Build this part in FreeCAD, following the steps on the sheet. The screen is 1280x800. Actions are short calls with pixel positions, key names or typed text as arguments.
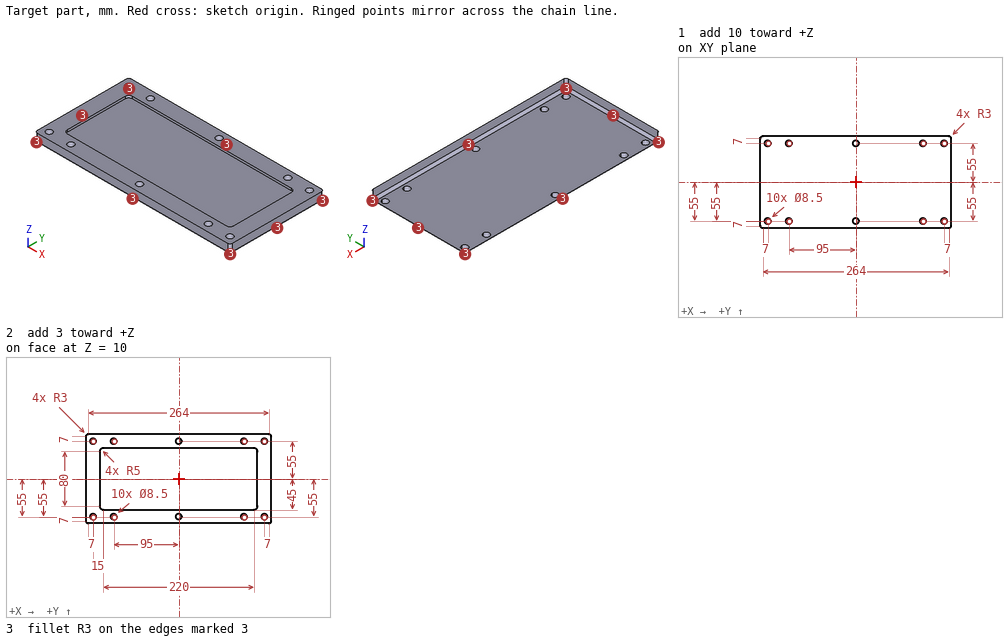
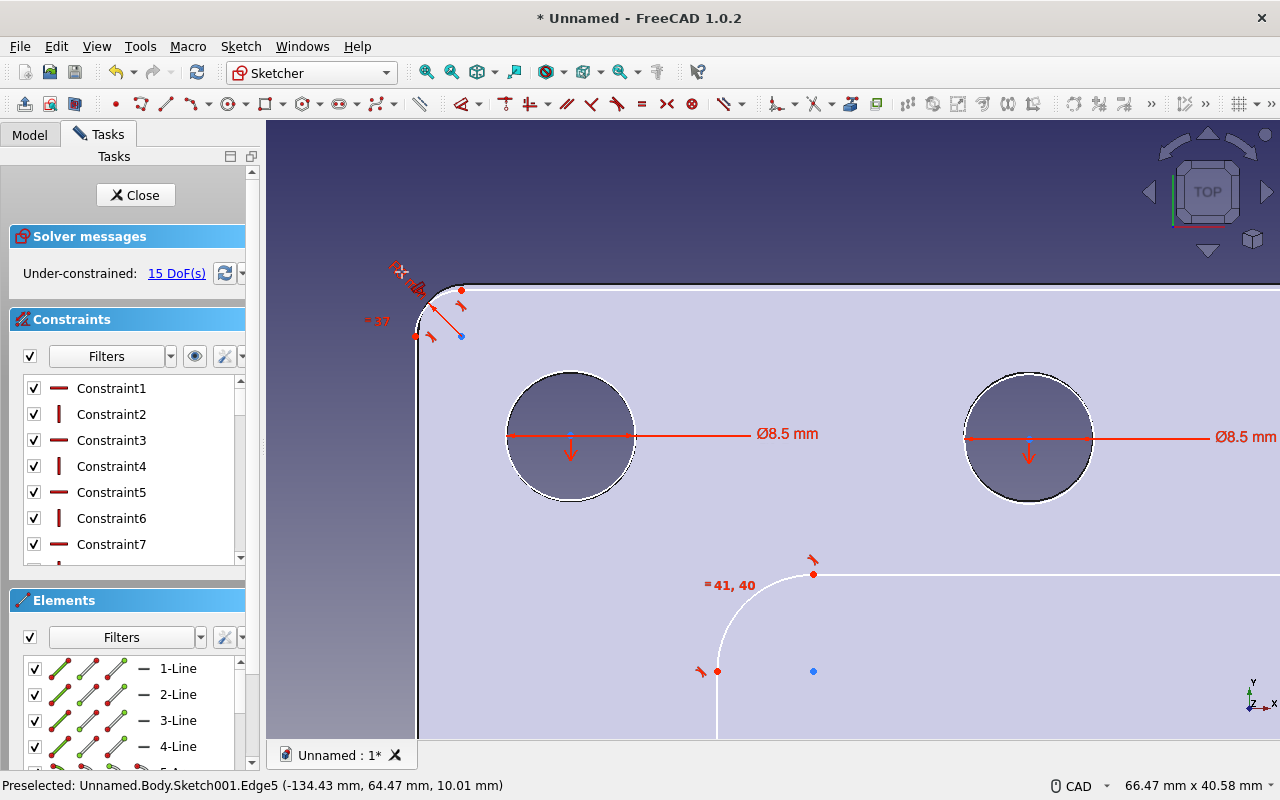
scroll(427, 297, down, 10)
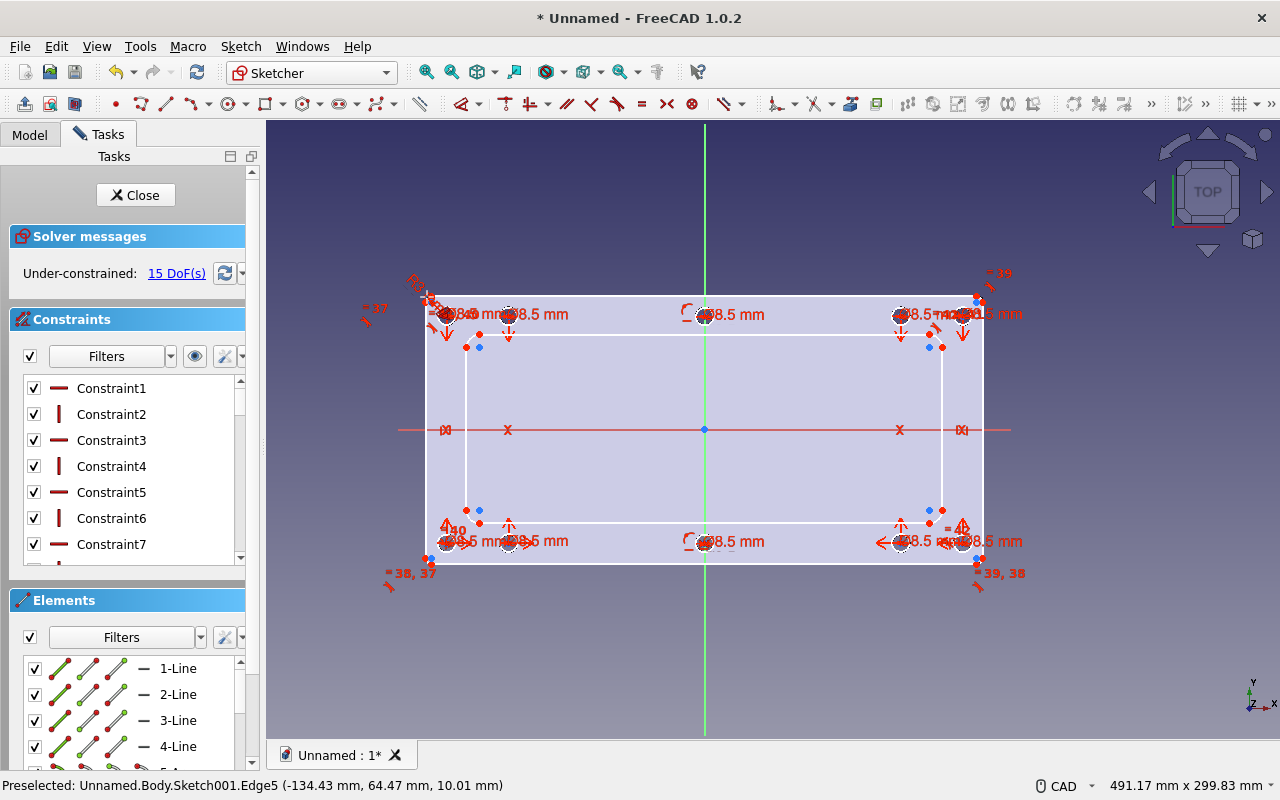
scroll(468, 516, up, 7)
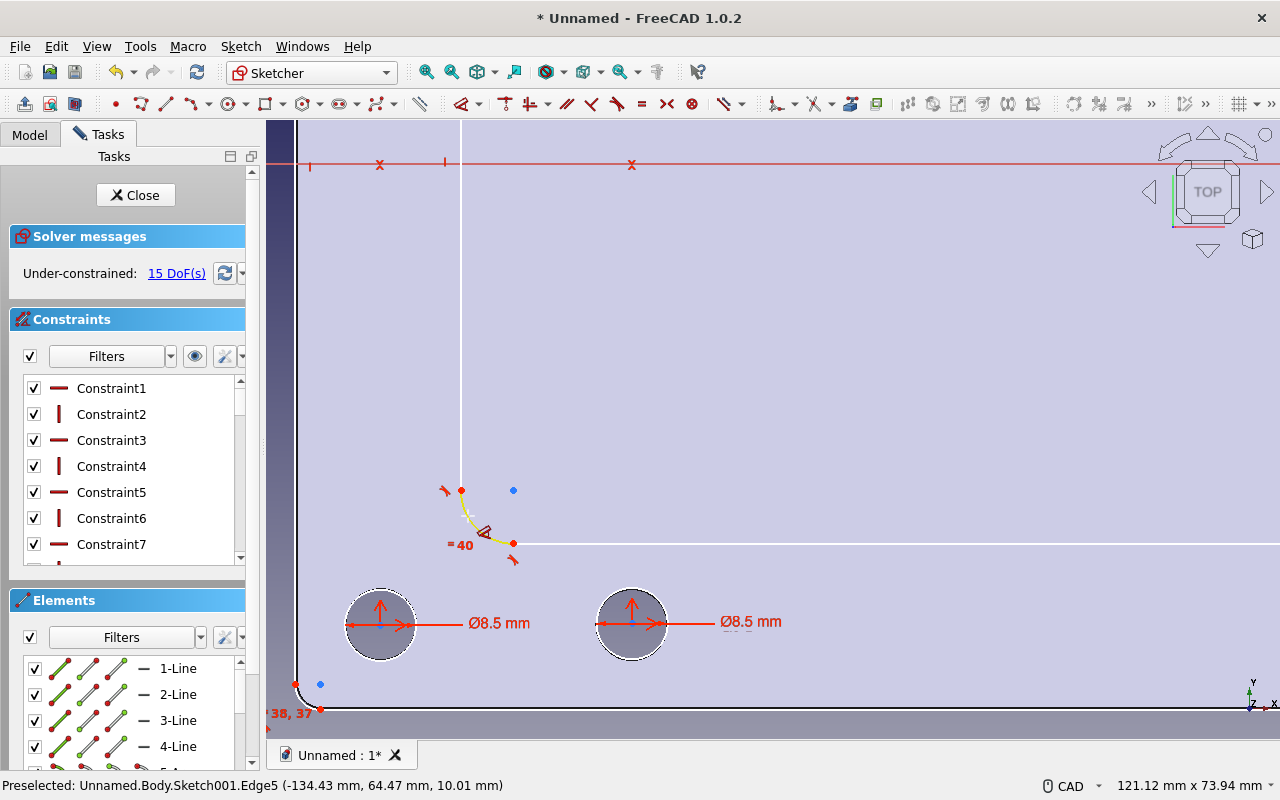
click(467, 515)
click(439, 530)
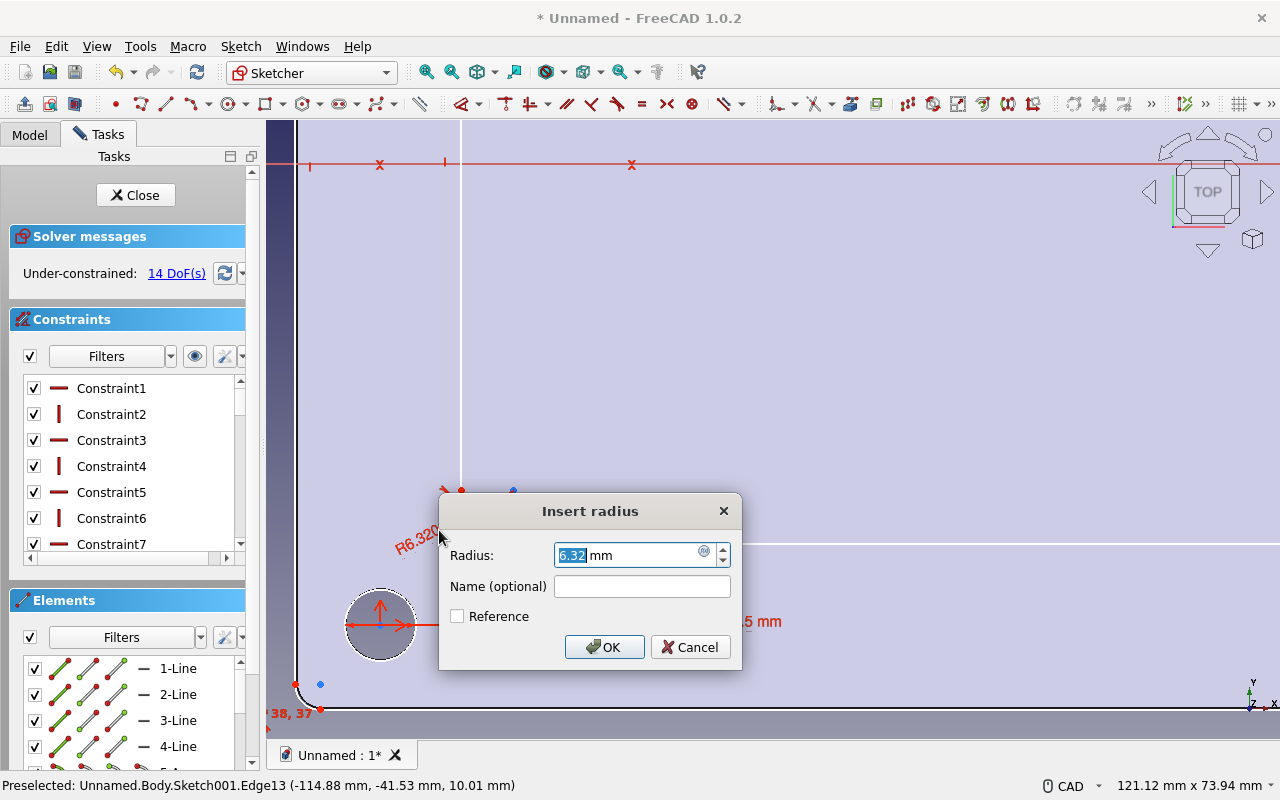
text(5)
key(Return)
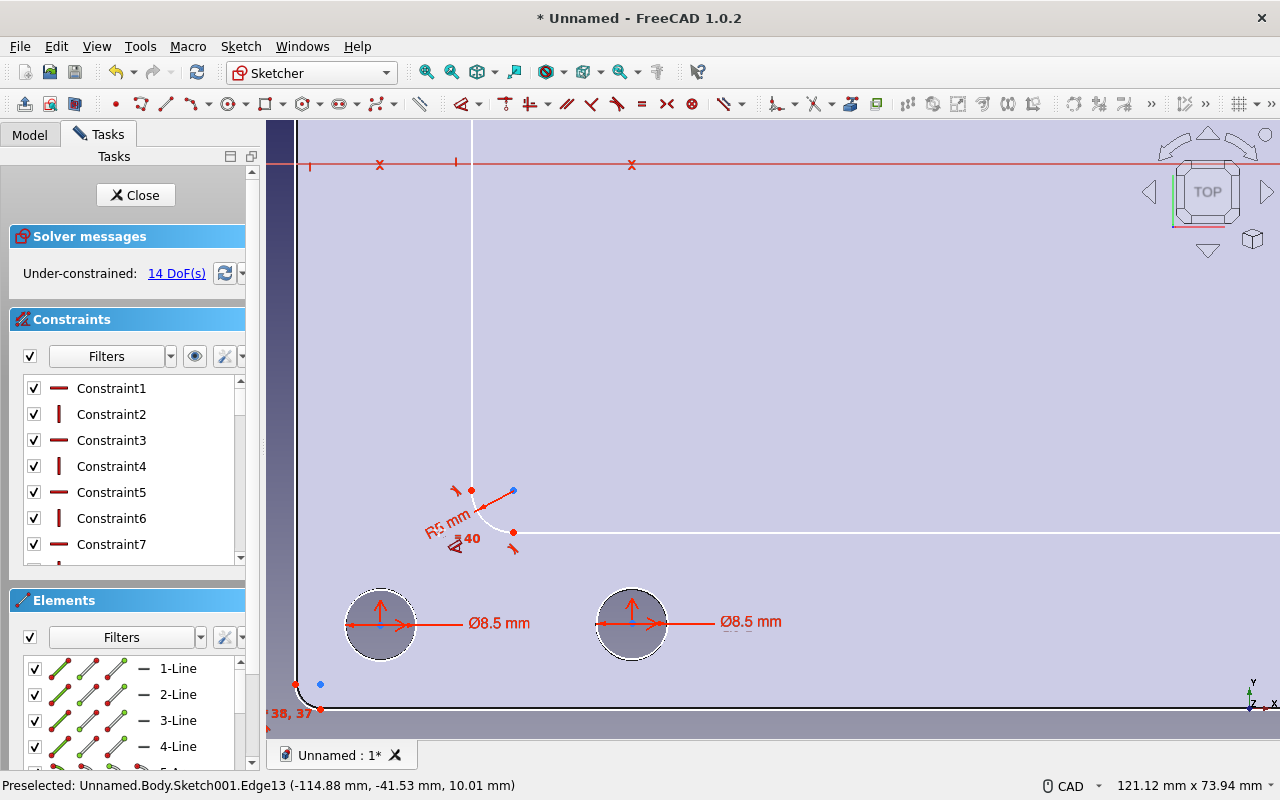
scroll(468, 516, down, 7)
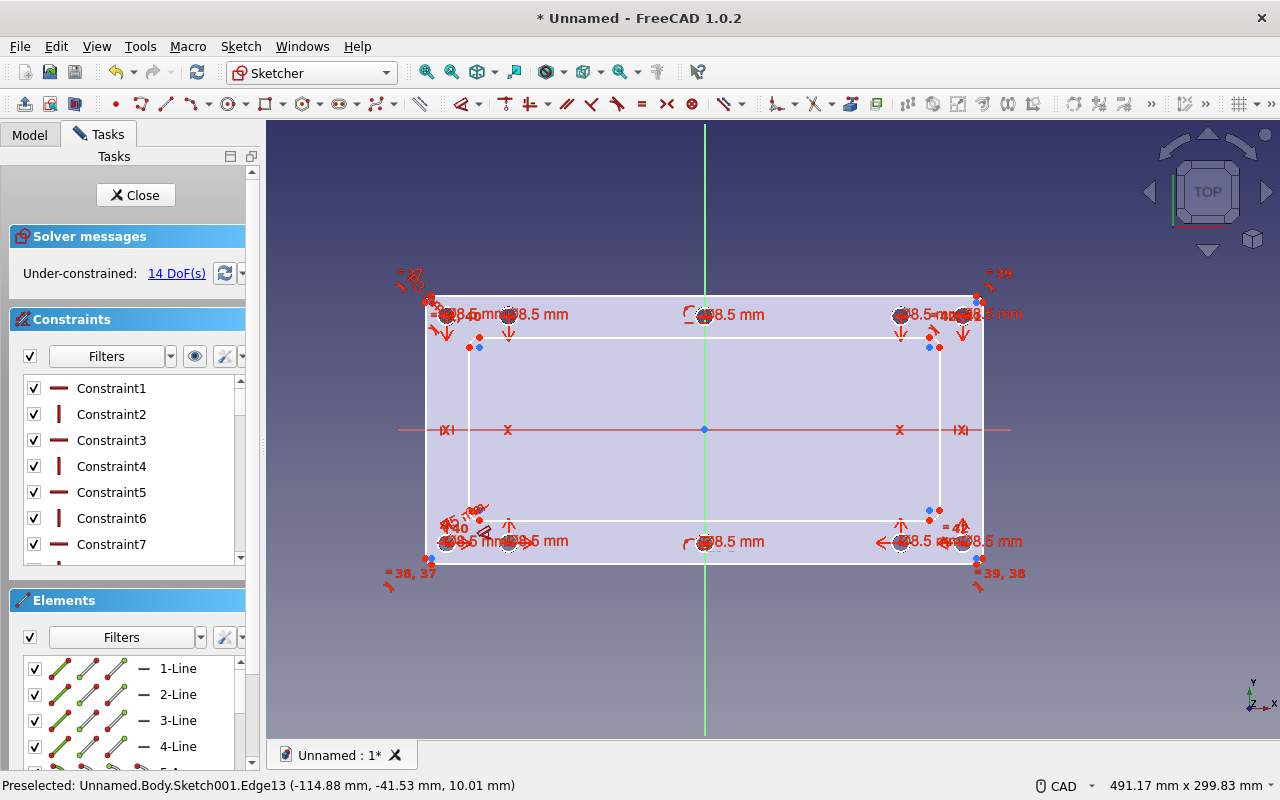
click(469, 462)
click(503, 392)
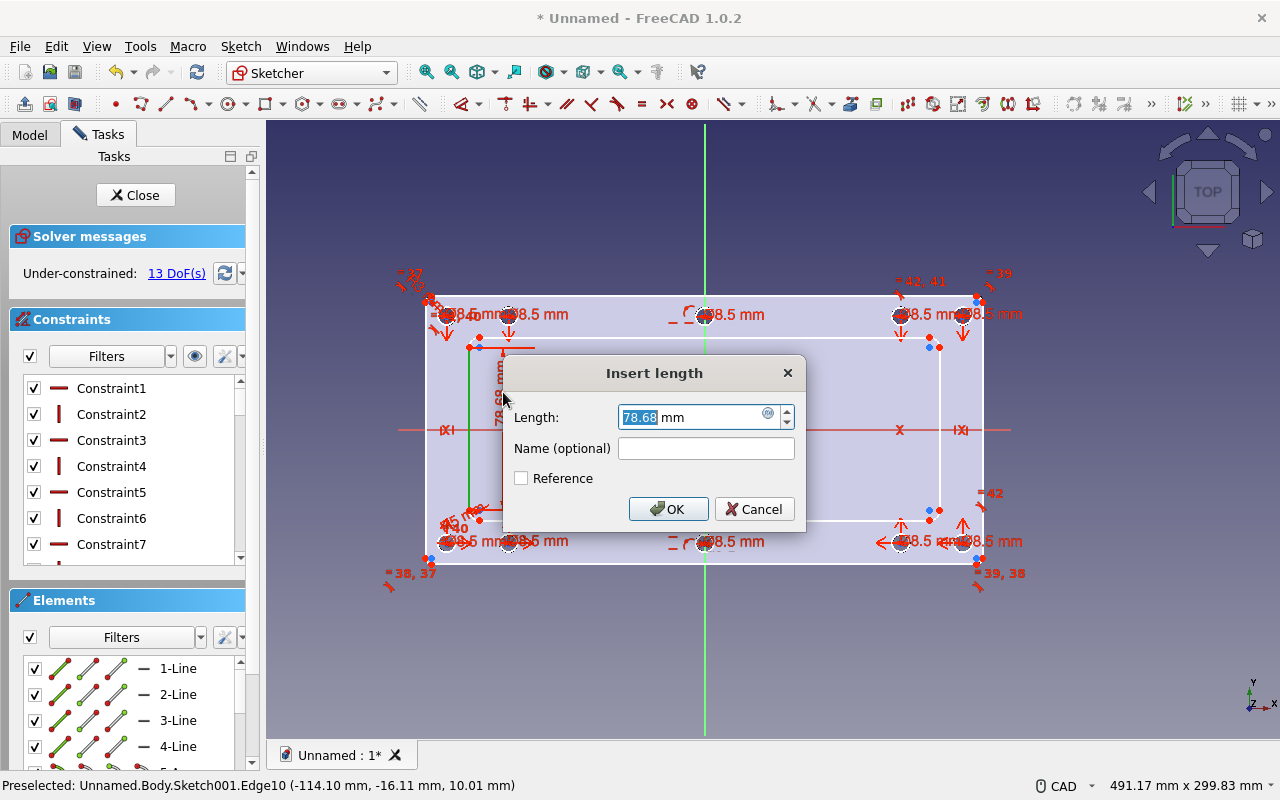
text(80)
key(Return)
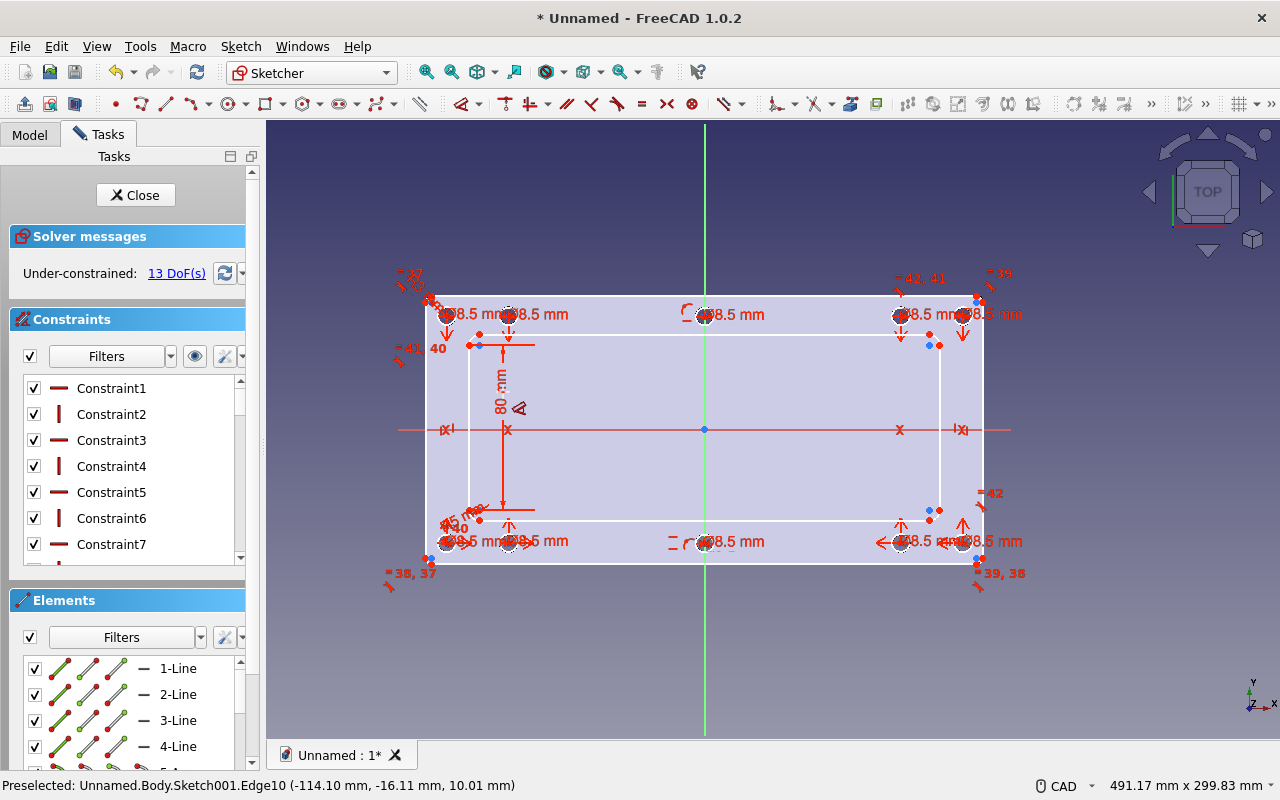
click(447, 543)
click(413, 487)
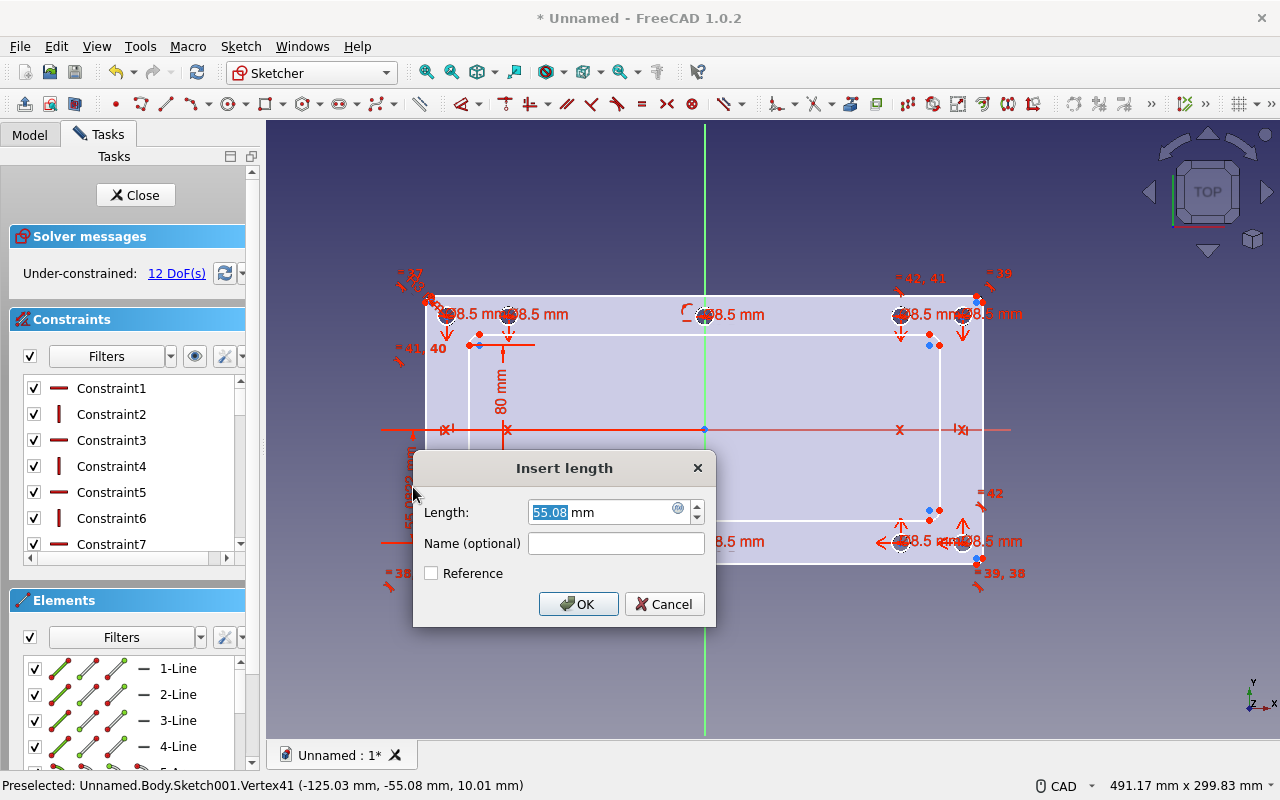
text(55)
key(Return)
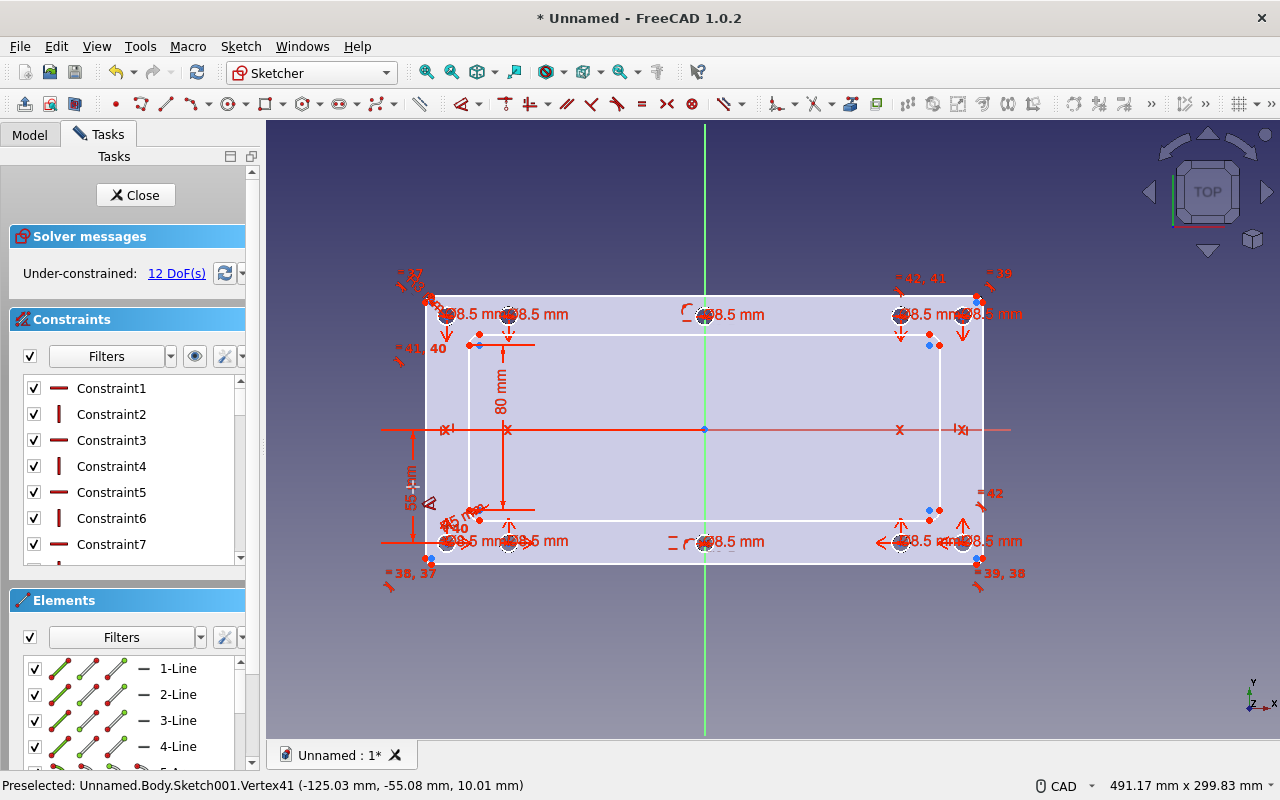
click(509, 543)
click(607, 396)